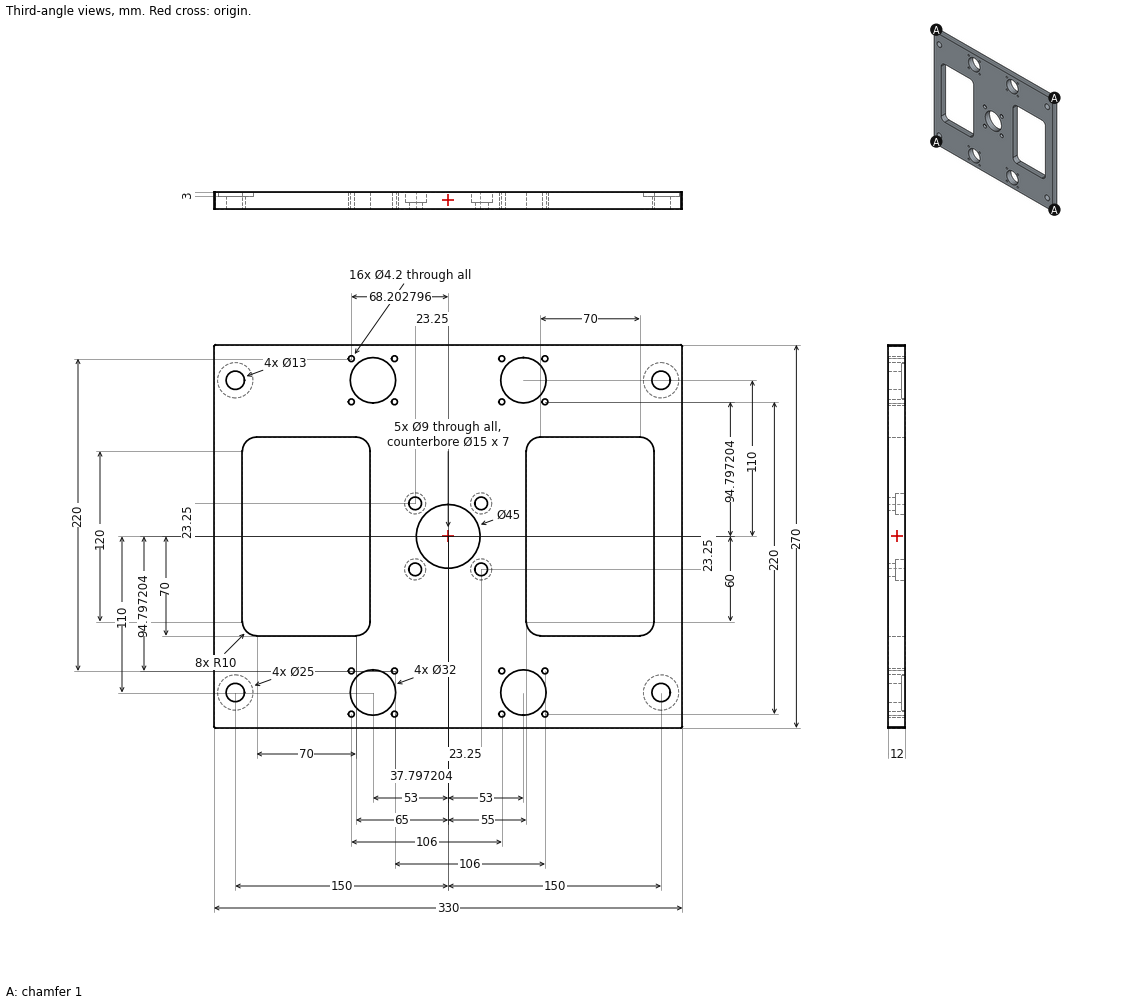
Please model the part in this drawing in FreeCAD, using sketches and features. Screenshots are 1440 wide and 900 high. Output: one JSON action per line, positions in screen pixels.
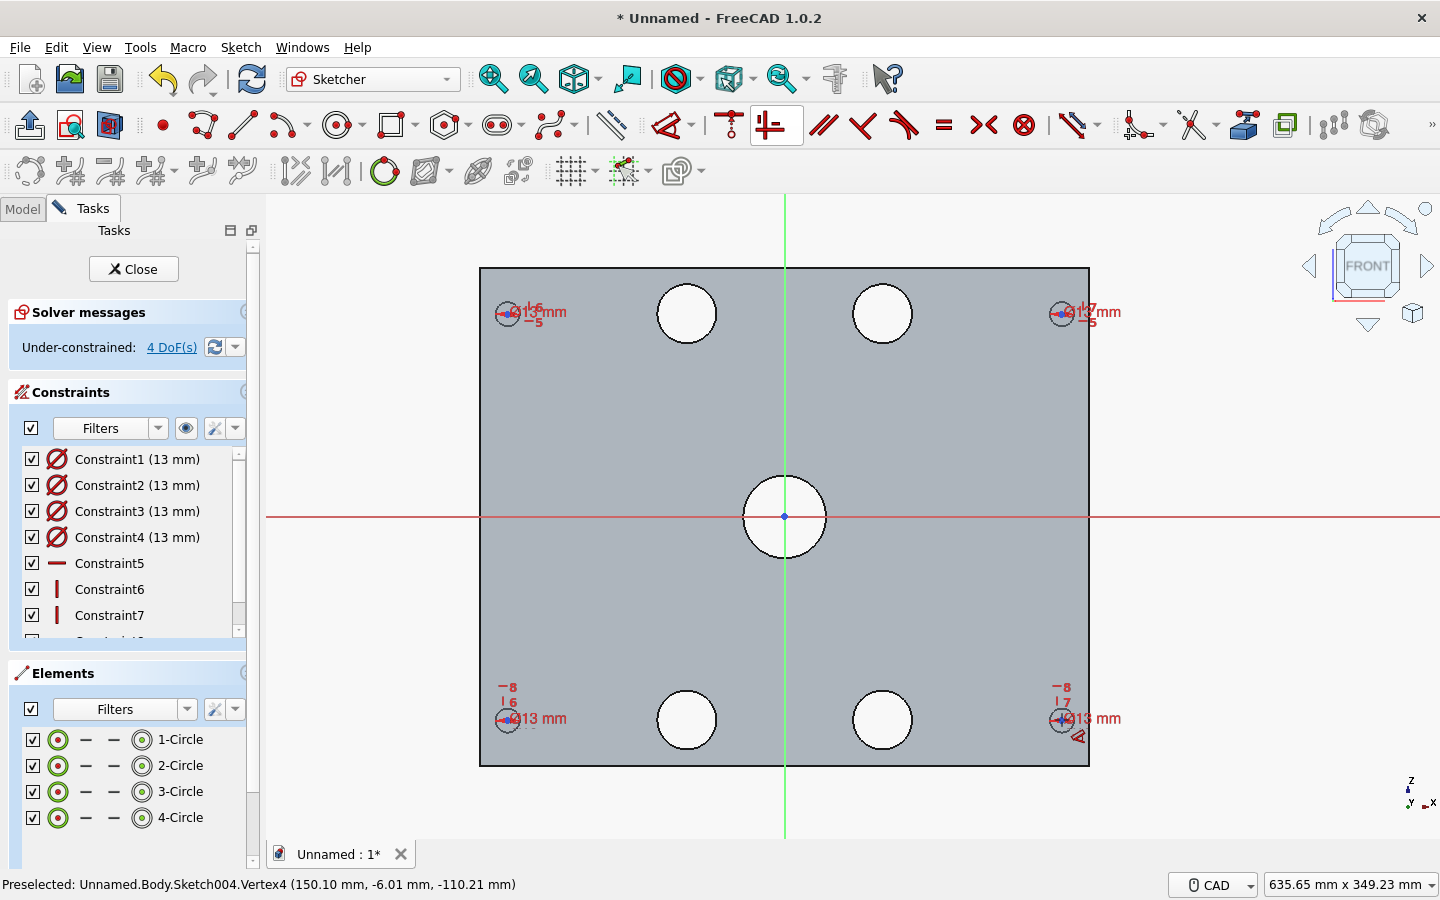
{"action": "left_click", "coordinate": [508, 314]}
{"action": "left_click", "coordinate": [646, 280]}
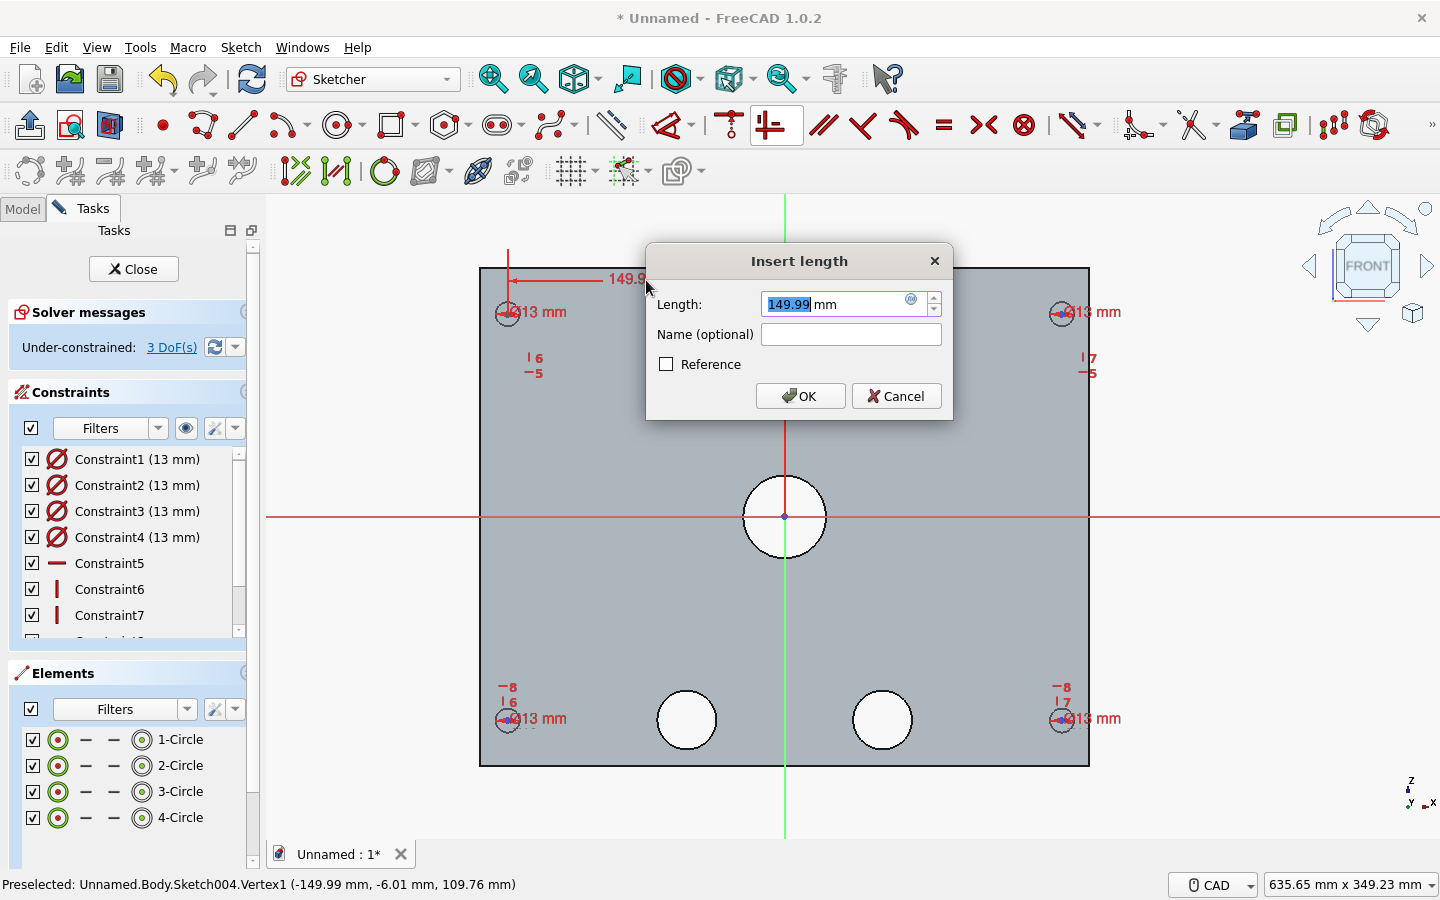
{"action": "type", "text": "150"}
{"action": "key", "text": "Return"}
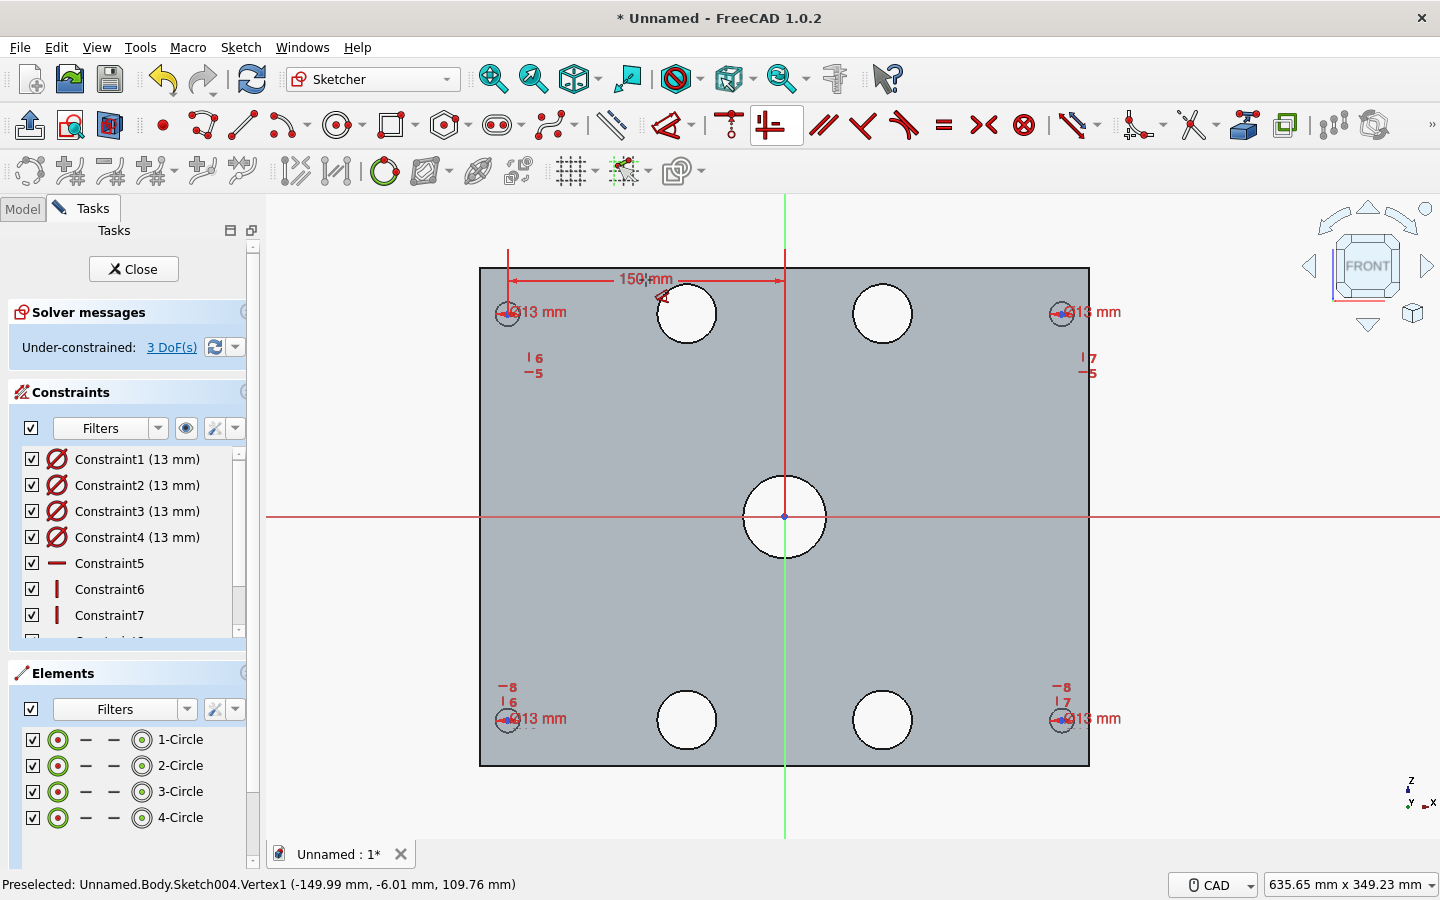
{"action": "left_click", "coordinate": [508, 314]}
{"action": "left_click", "coordinate": [474, 416]}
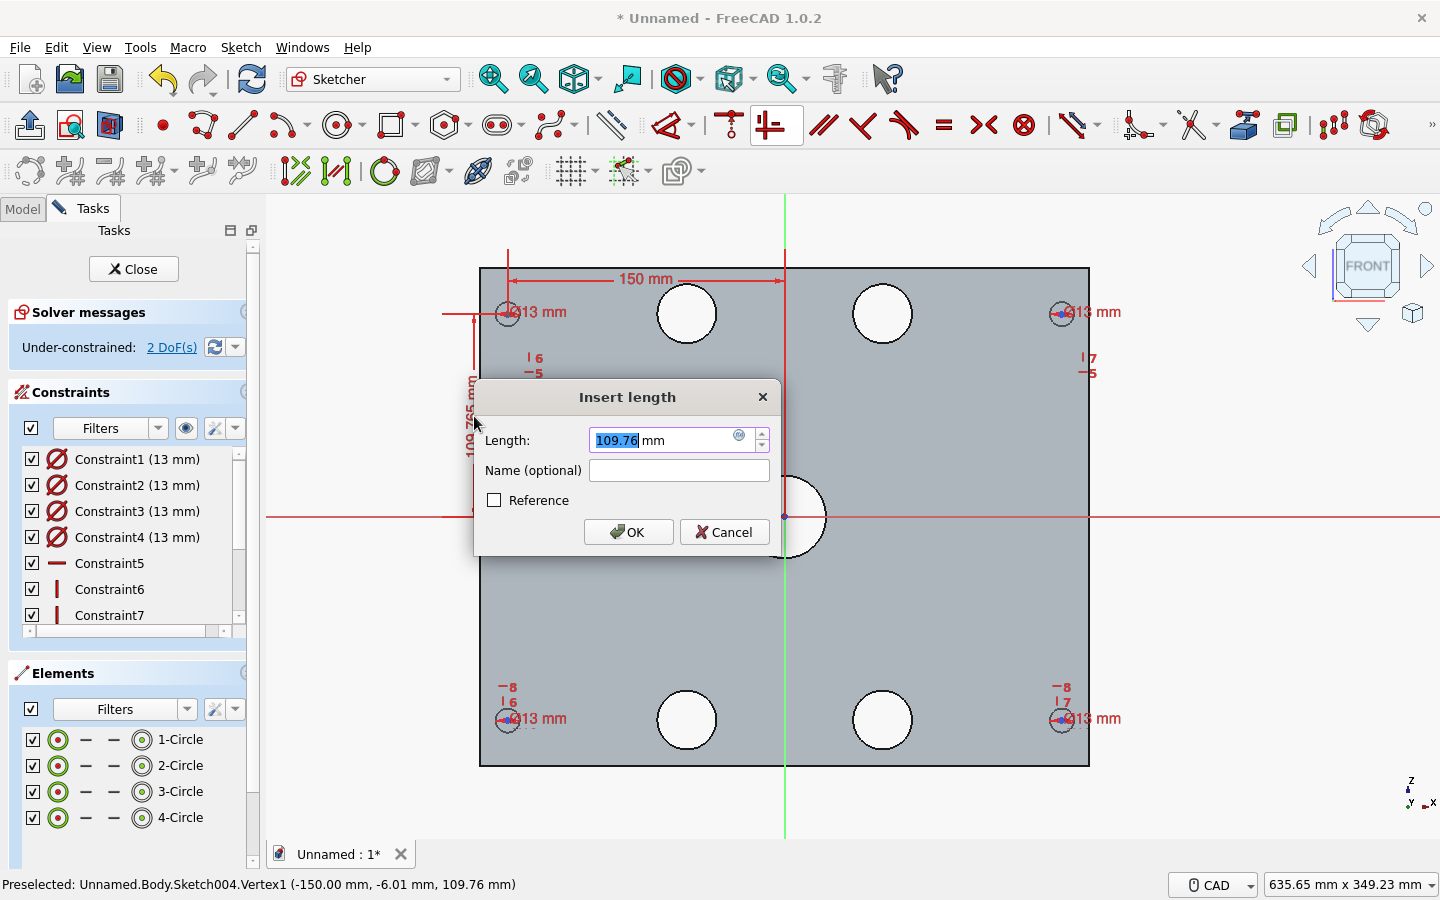
{"action": "type", "text": "110"}
{"action": "key", "text": "Return"}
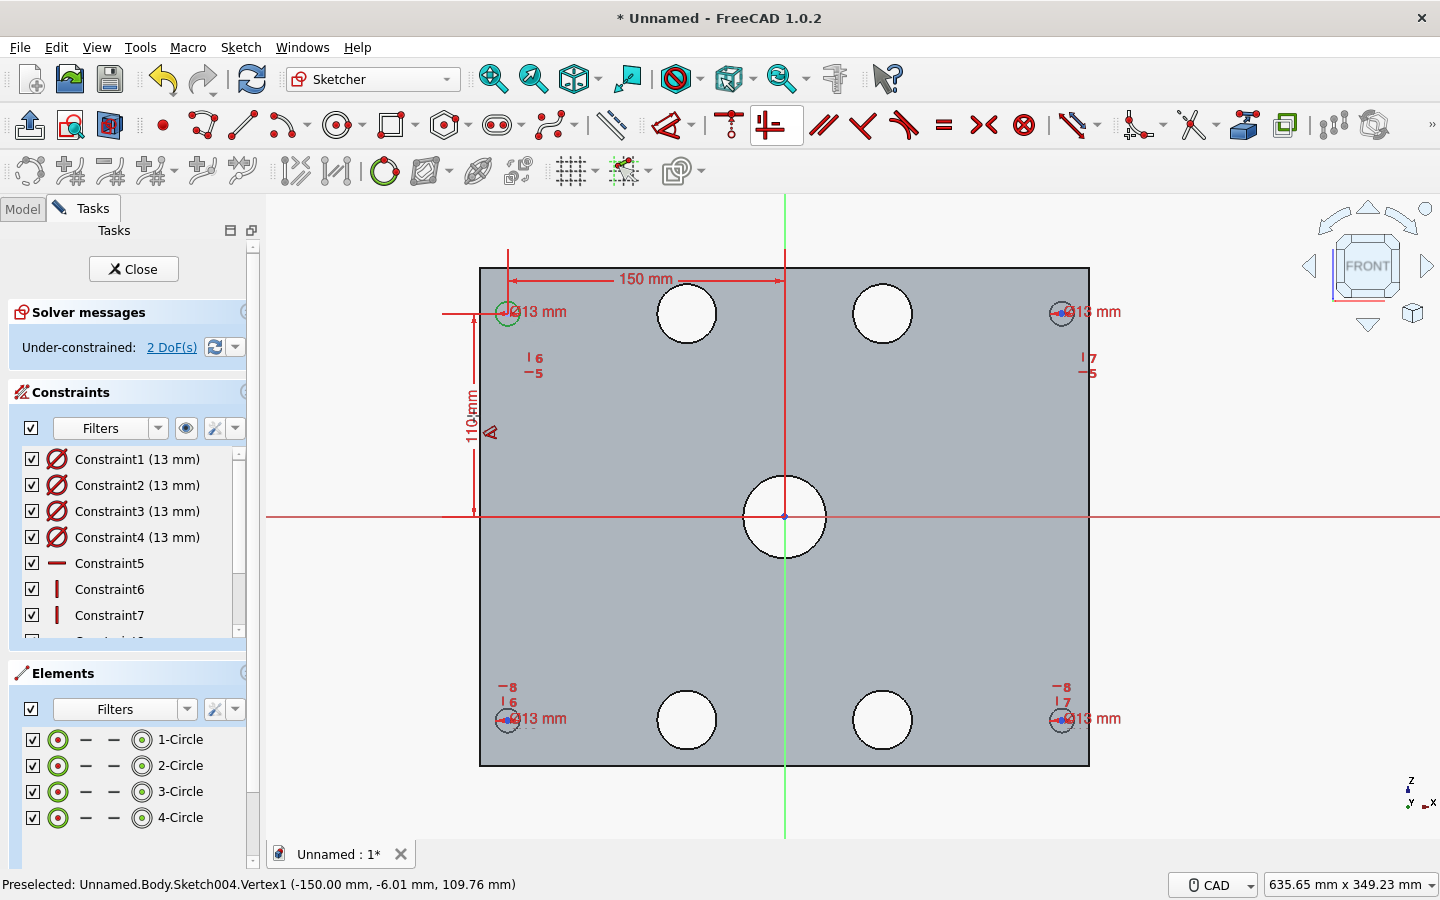
{"action": "left_click", "coordinate": [1062, 314]}
{"action": "left_click", "coordinate": [923, 280]}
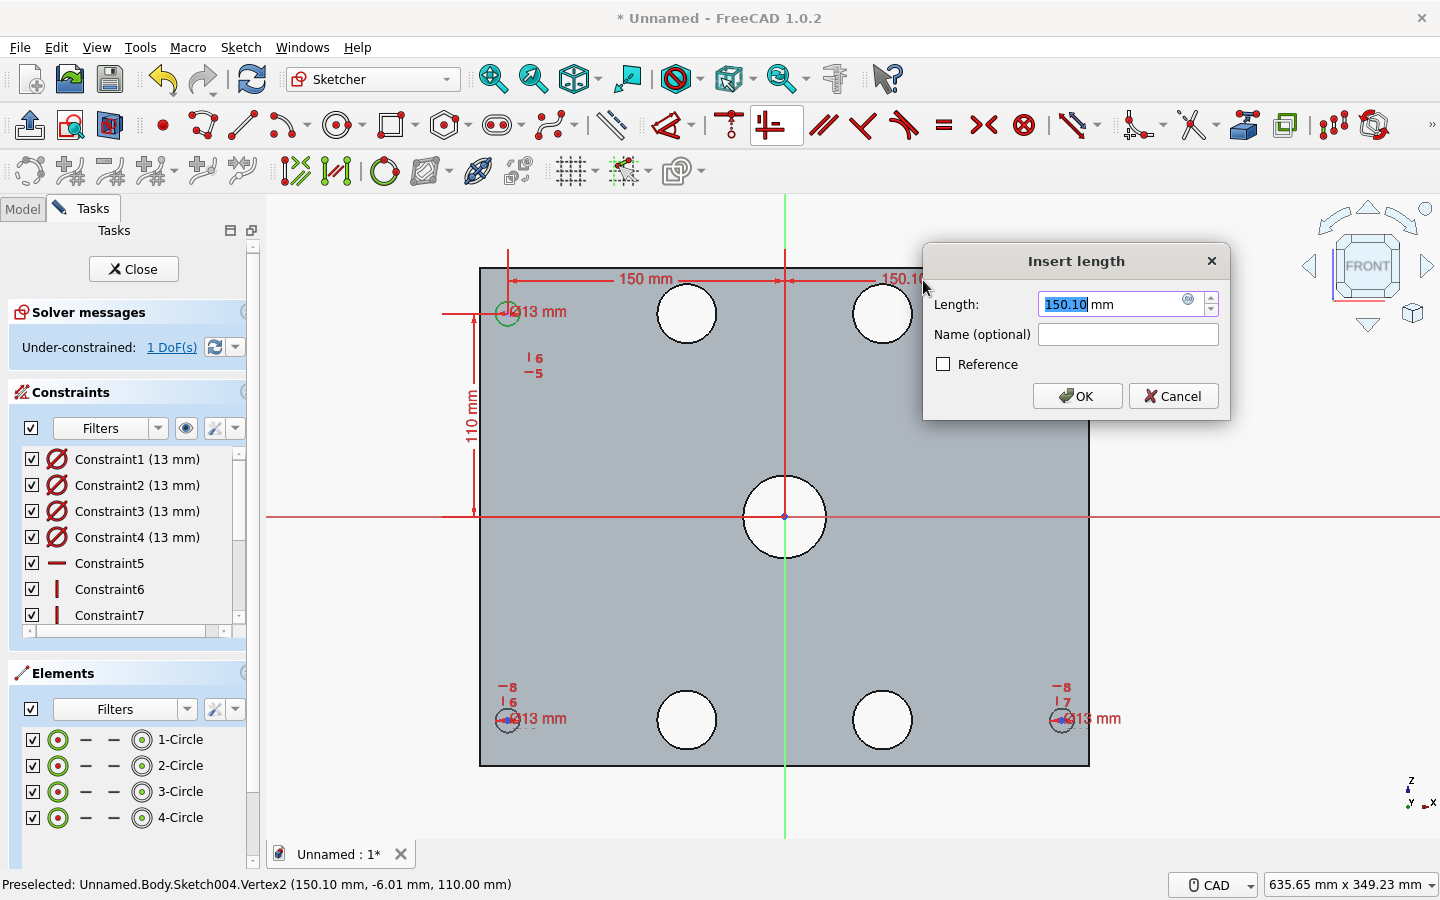
{"action": "type", "text": "150"}
{"action": "key", "text": "Return"}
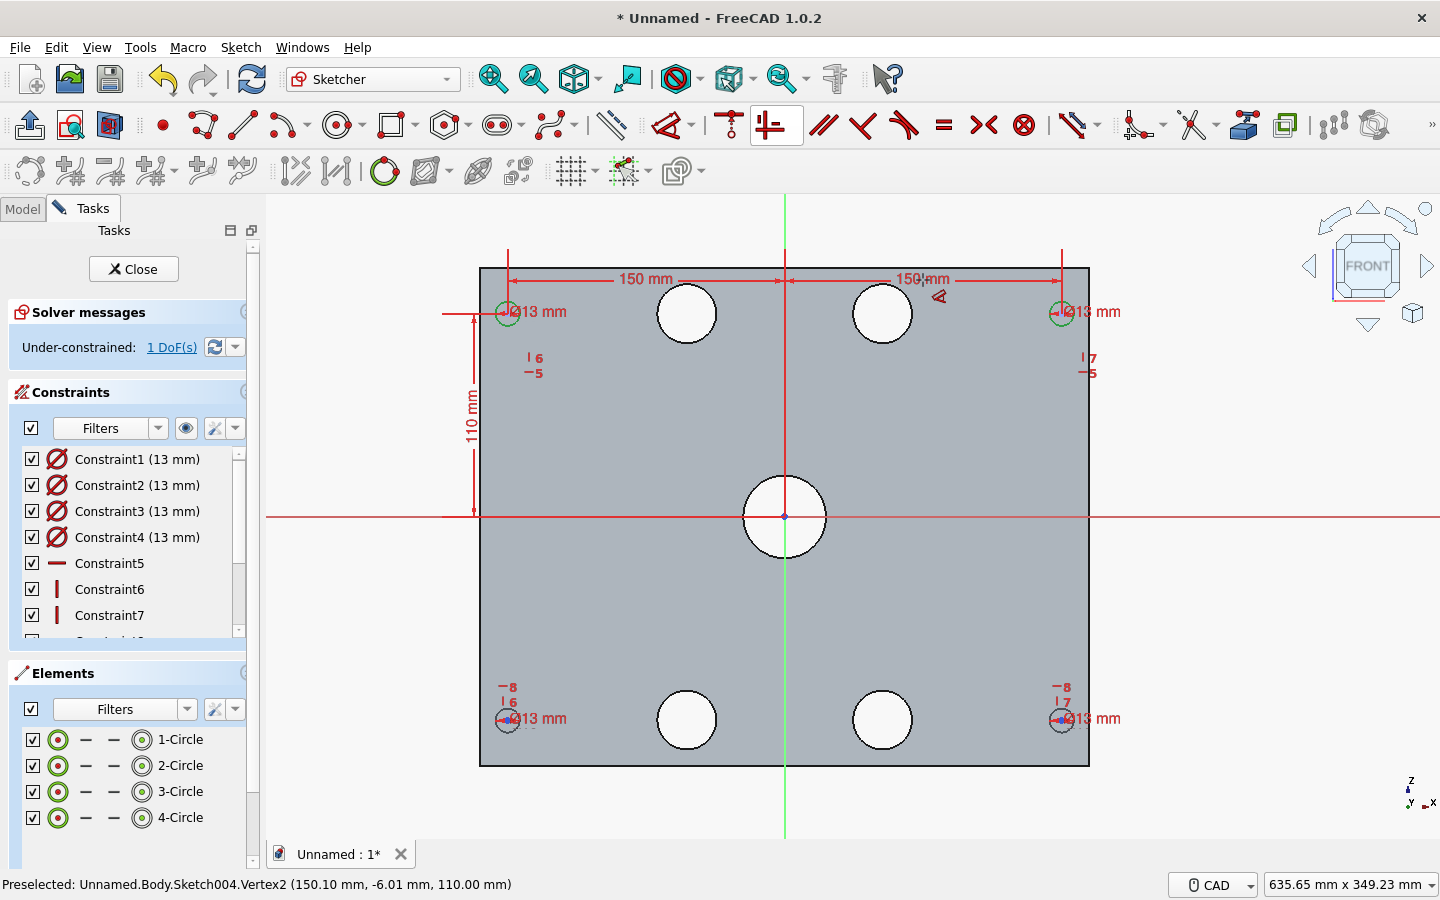
{"action": "left_click", "coordinate": [508, 721]}
{"action": "left_click", "coordinate": [474, 619]}